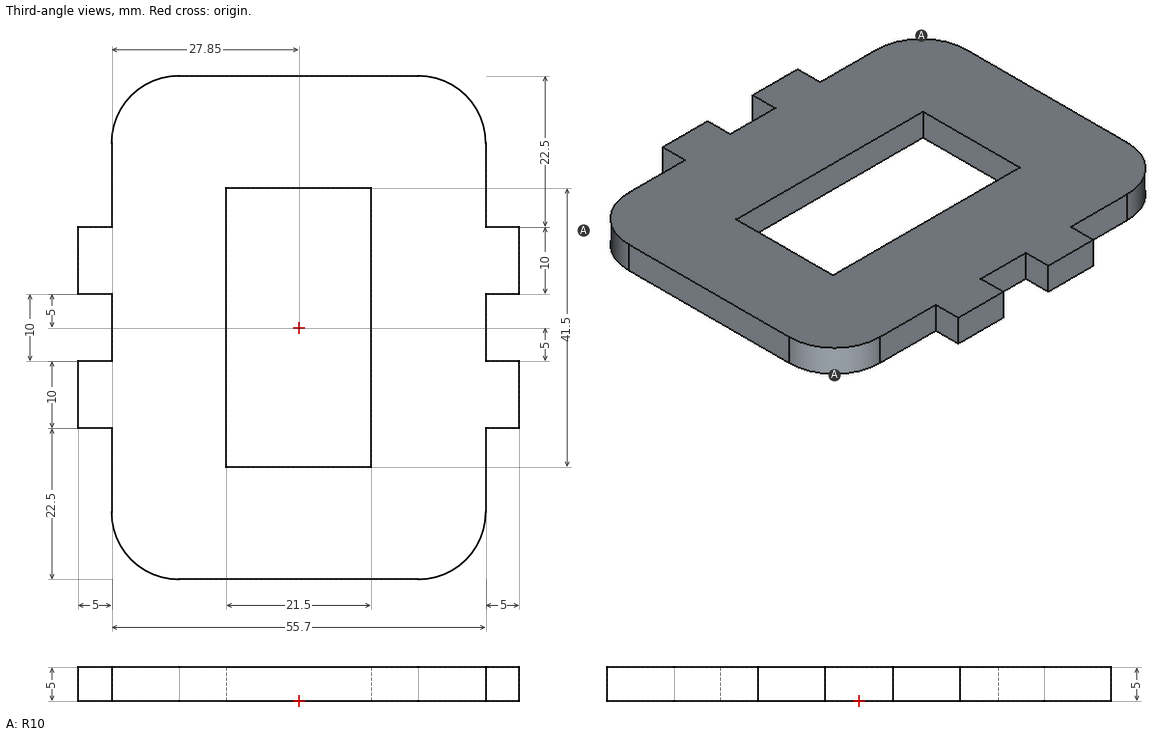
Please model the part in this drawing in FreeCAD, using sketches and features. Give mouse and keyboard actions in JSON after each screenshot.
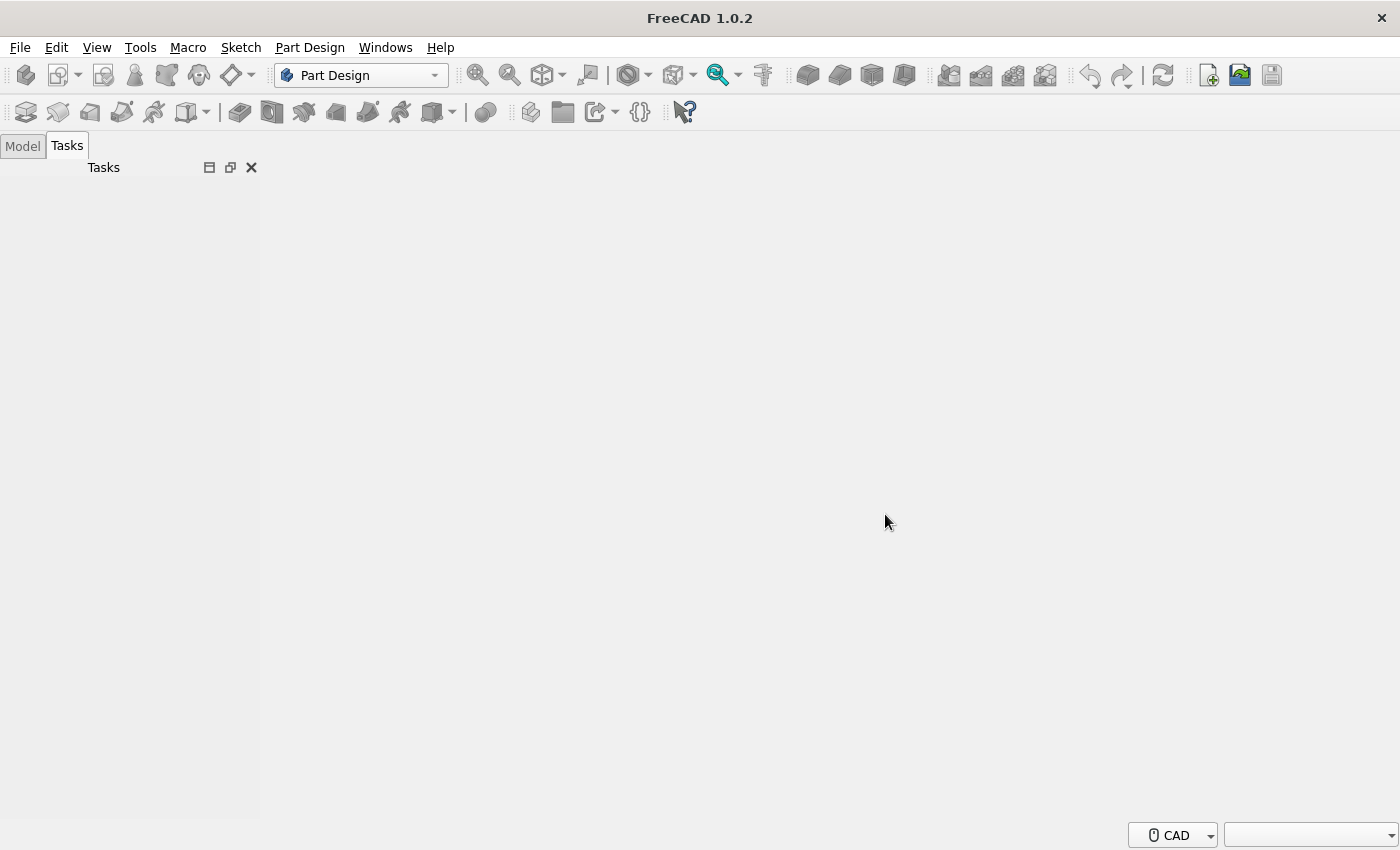
{"action": "key", "text": "ctrl+n"}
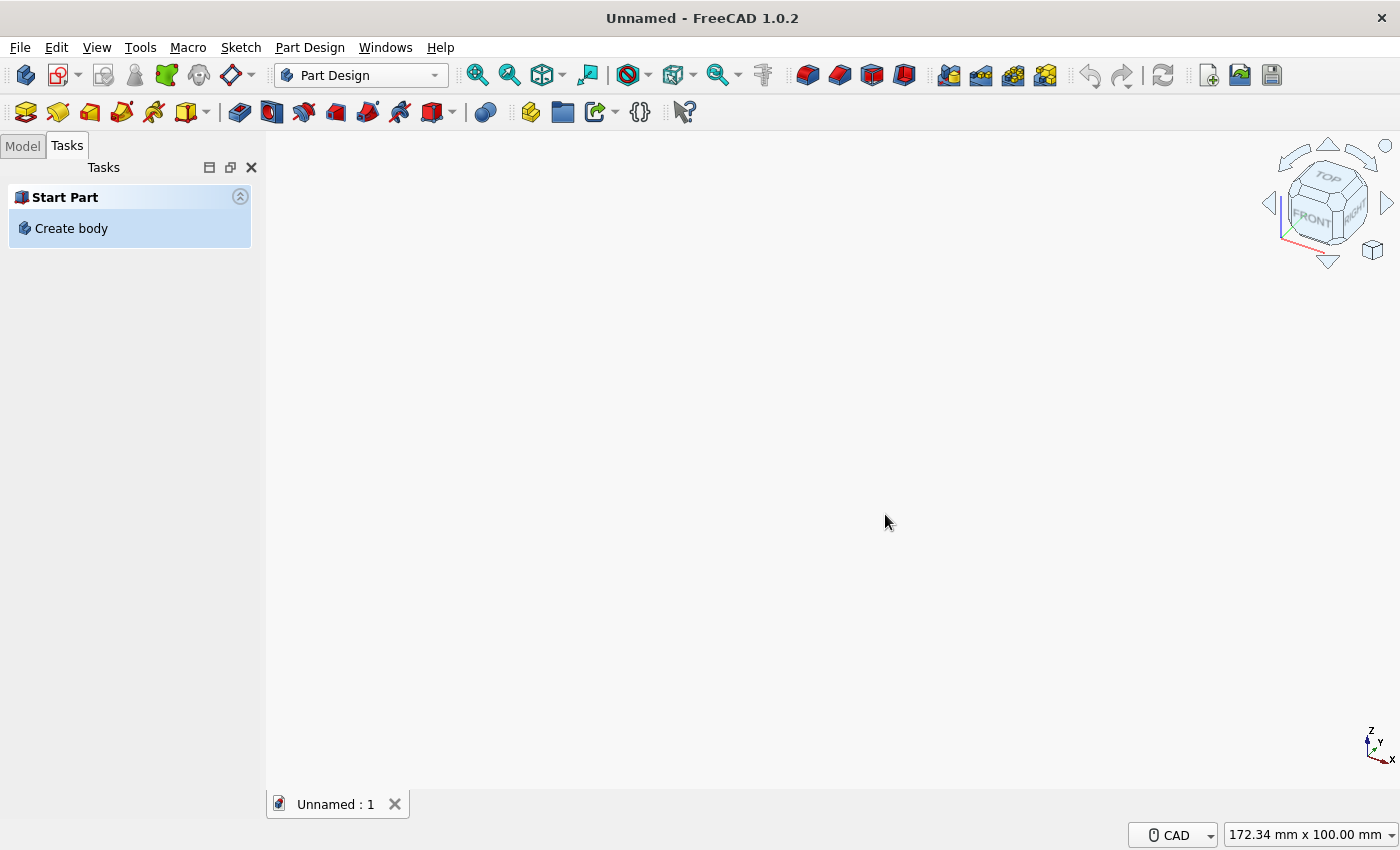
{"action": "left_click", "coordinate": [58, 76]}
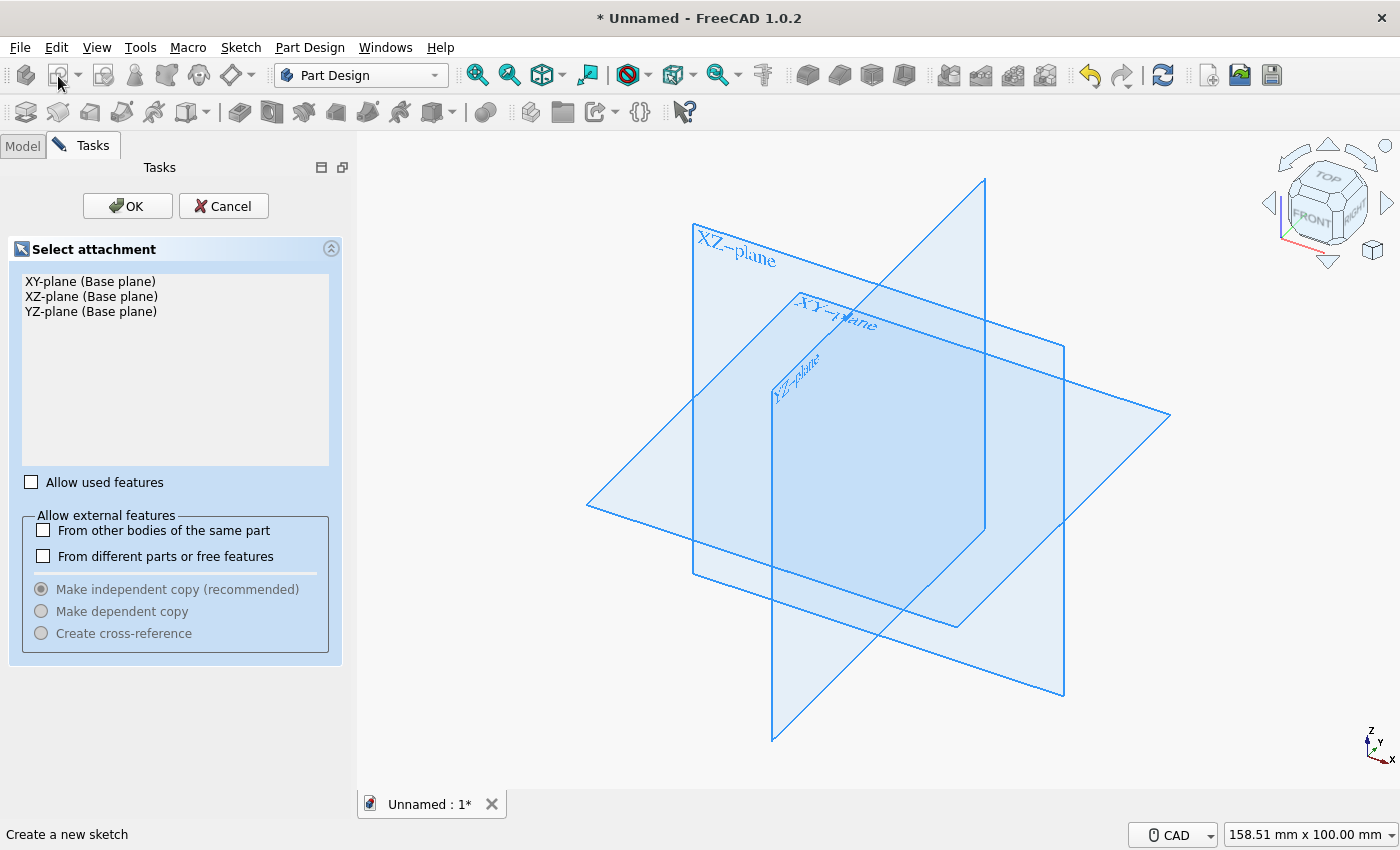
{"action": "left_click", "coordinate": [82, 282]}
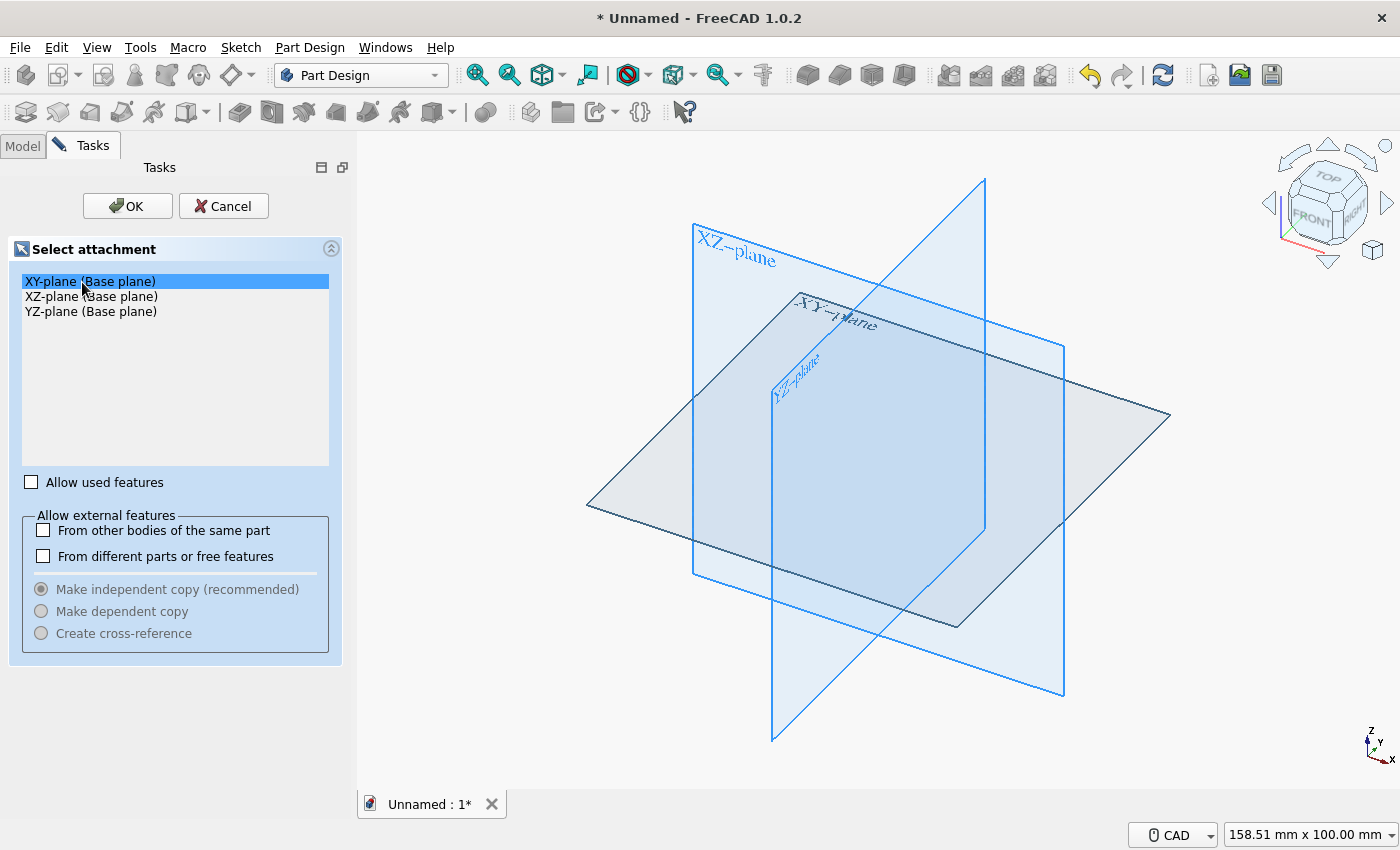
{"action": "left_click", "coordinate": [128, 206]}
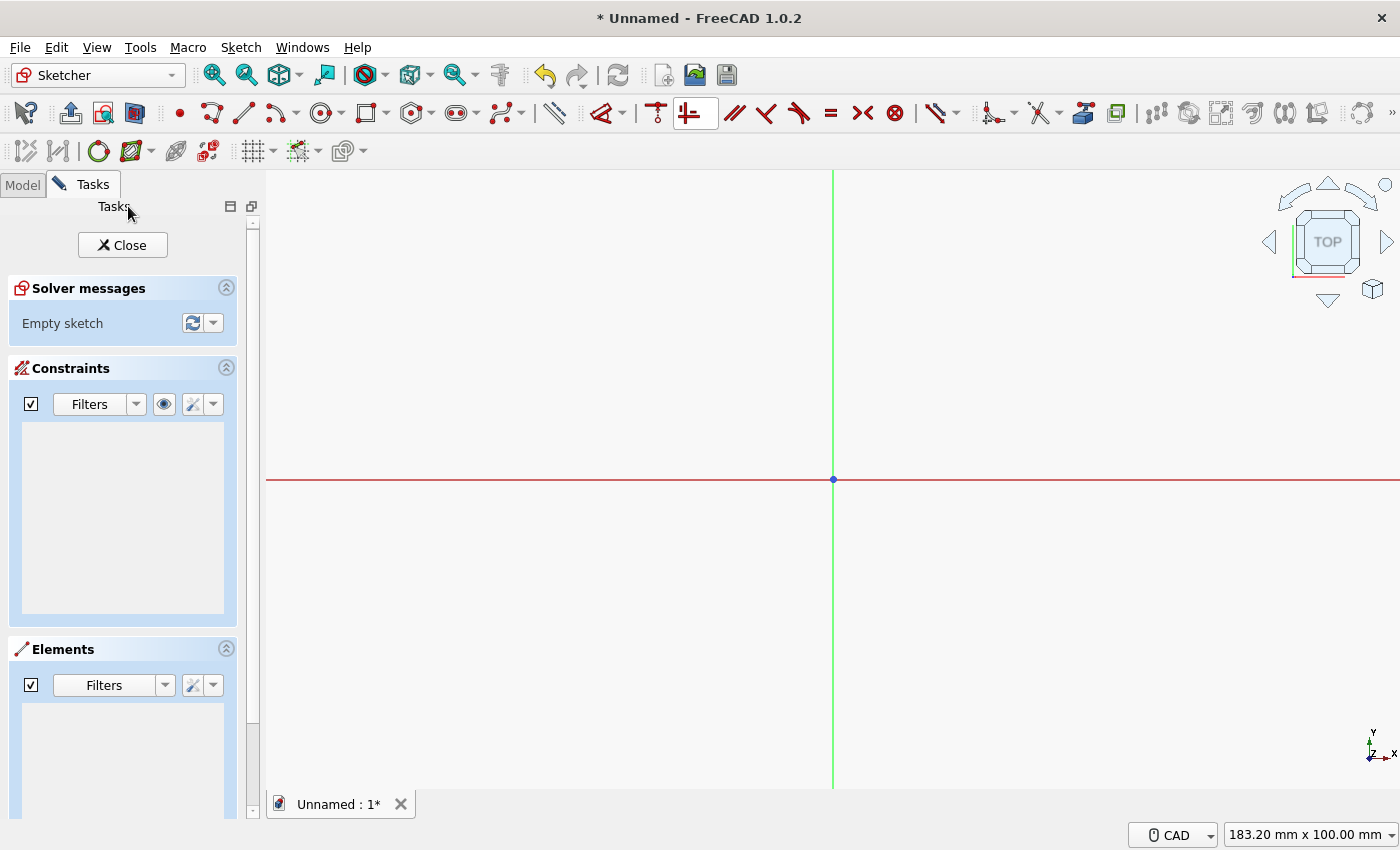
{"action": "left_click", "coordinate": [212, 114]}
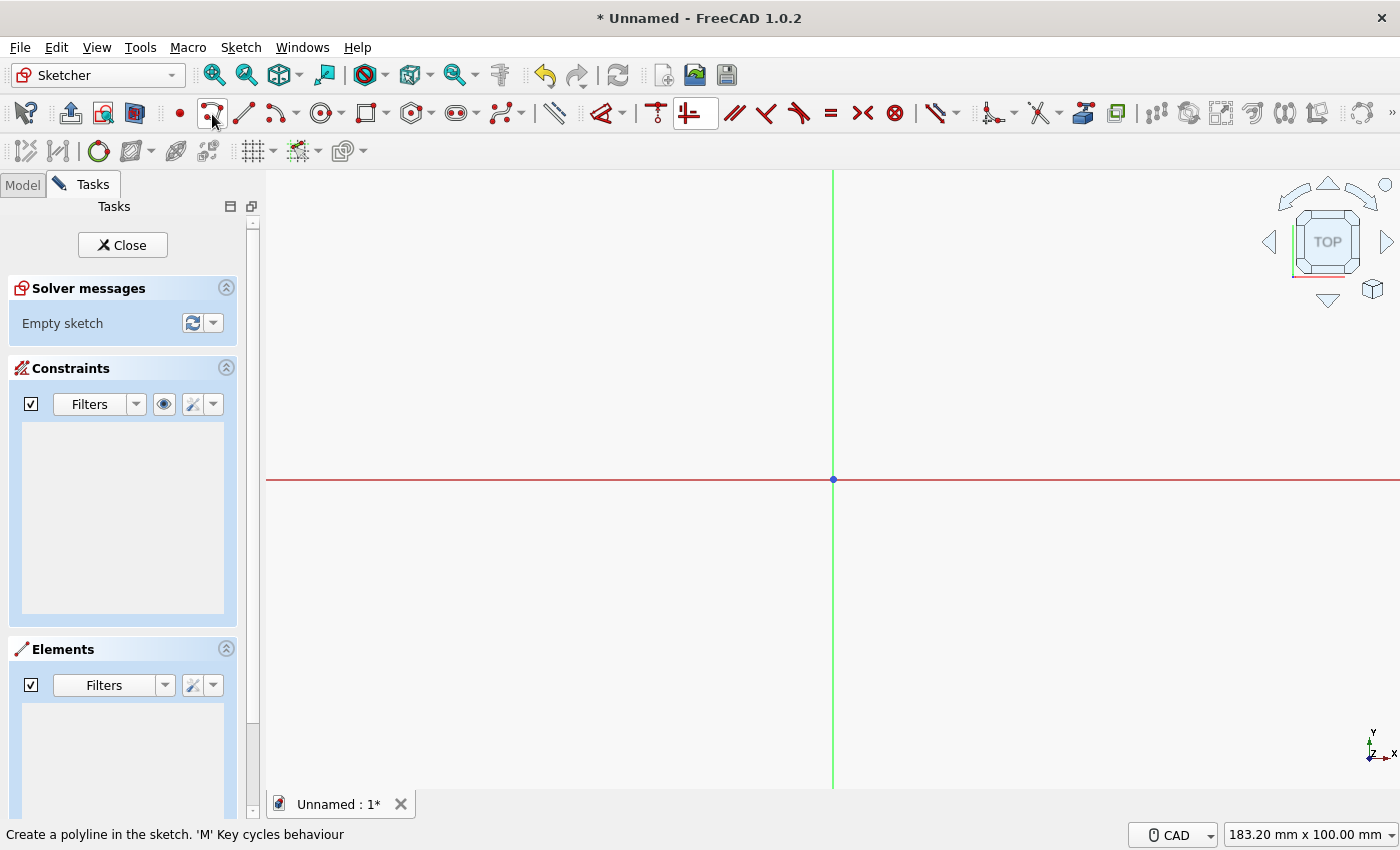
{"action": "left_click", "coordinate": [661, 449]}
{"action": "left_click", "coordinate": [661, 510]}
{"action": "left_click", "coordinate": [630, 510]}
{"action": "left_click", "coordinate": [630, 572]}
{"action": "left_click", "coordinate": [661, 572]}
{"action": "left_click", "coordinate": [661, 712]}
{"action": "left_click", "coordinate": [1005, 712]}
{"action": "left_click", "coordinate": [1005, 572]}
{"action": "left_click", "coordinate": [1036, 572]}
{"action": "left_click", "coordinate": [1036, 510]}
{"action": "left_click", "coordinate": [1005, 510]}
{"action": "left_click", "coordinate": [1005, 449]}
{"action": "left_click", "coordinate": [1036, 449]}
{"action": "left_click", "coordinate": [1036, 387]}
{"action": "left_click", "coordinate": [1005, 387]}
{"action": "left_click", "coordinate": [1005, 247]}
{"action": "left_click", "coordinate": [661, 247]}
{"action": "left_click", "coordinate": [661, 387]}
{"action": "left_click", "coordinate": [630, 387]}
{"action": "left_click", "coordinate": [630, 449]}
{"action": "left_click", "coordinate": [661, 450]}
{"action": "key", "text": "Escape"}
{"action": "key", "text": "Escape"}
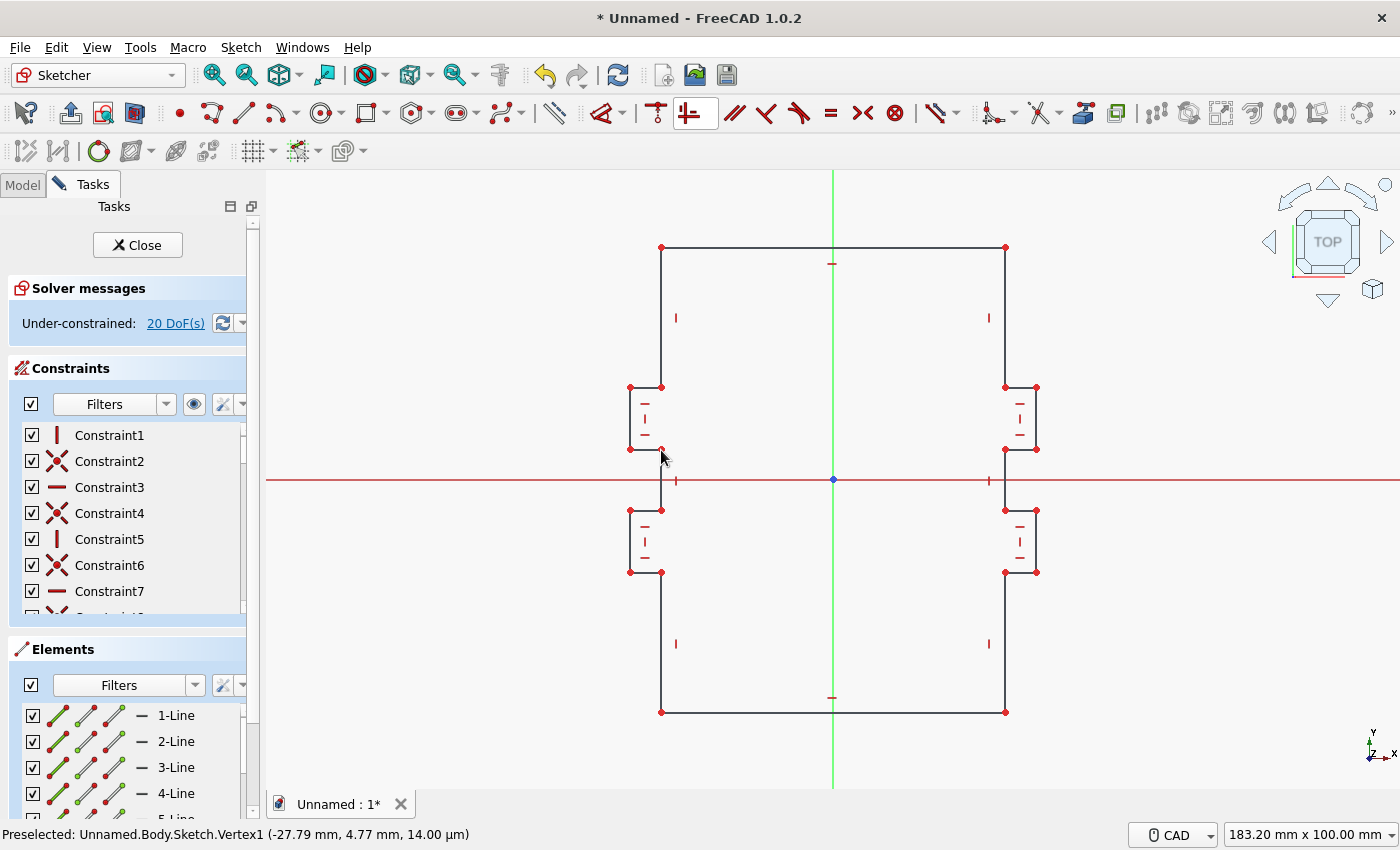
{"action": "scroll", "coordinate": [652, 511], "scroll_direction": "up", "scroll_amount": 2}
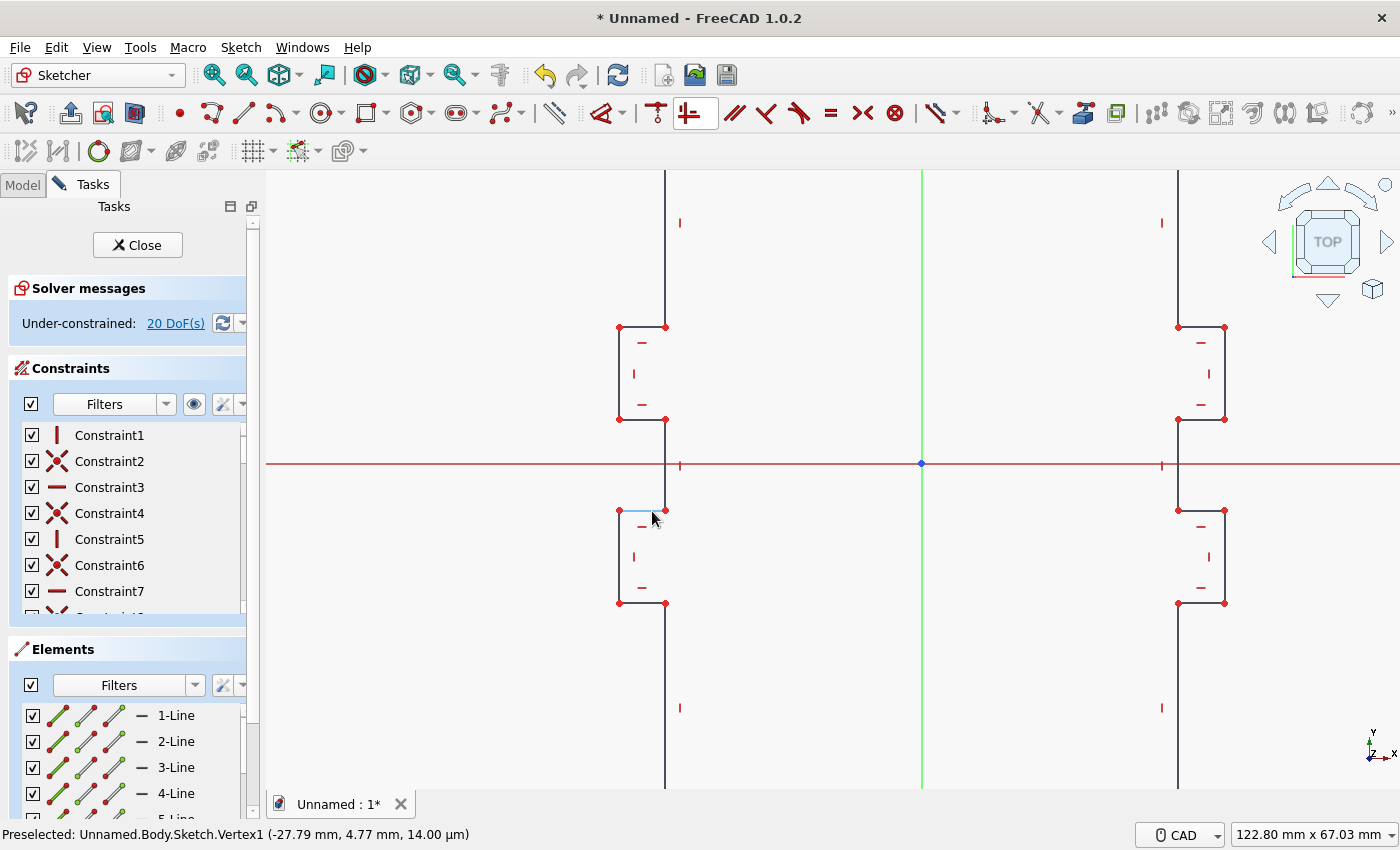
{"action": "left_click", "coordinate": [651, 511]}